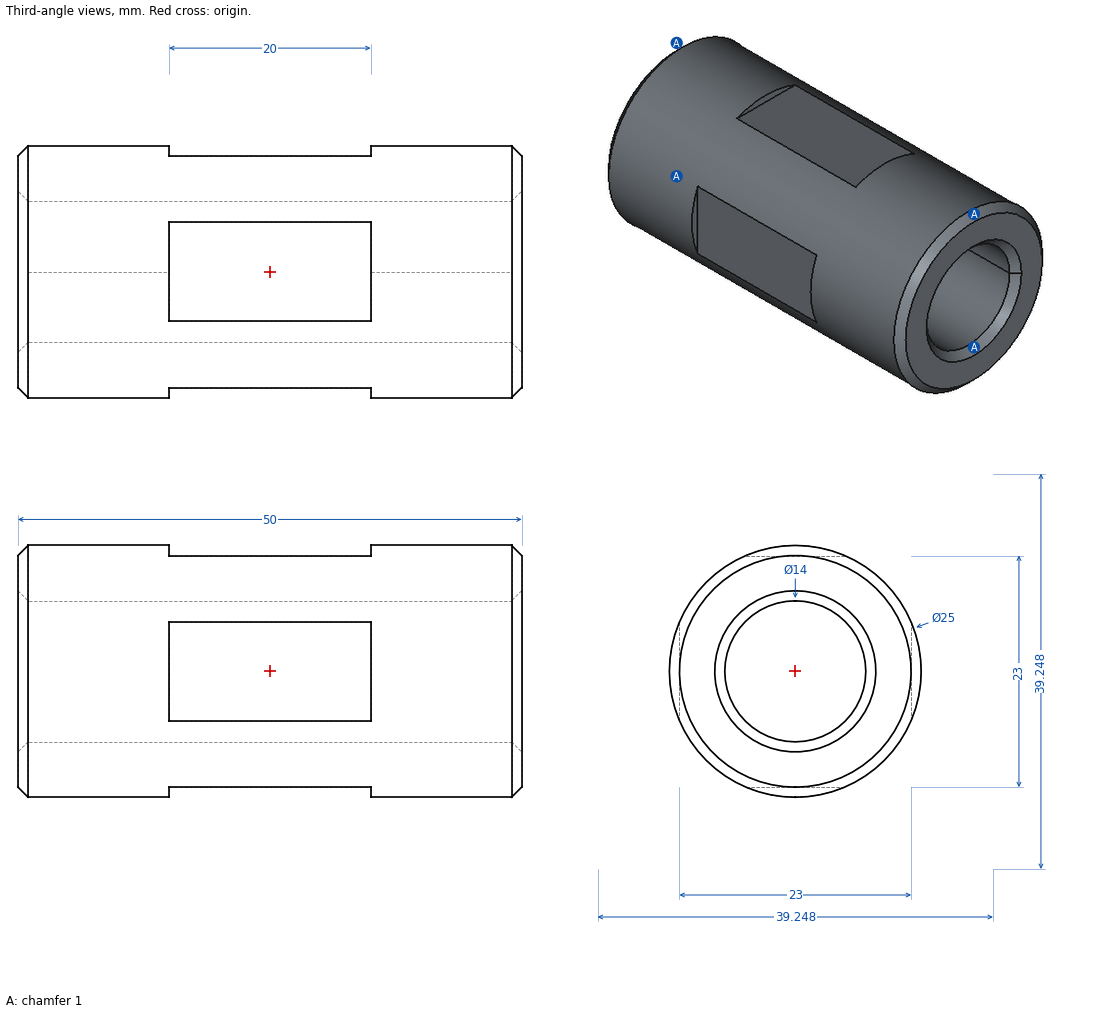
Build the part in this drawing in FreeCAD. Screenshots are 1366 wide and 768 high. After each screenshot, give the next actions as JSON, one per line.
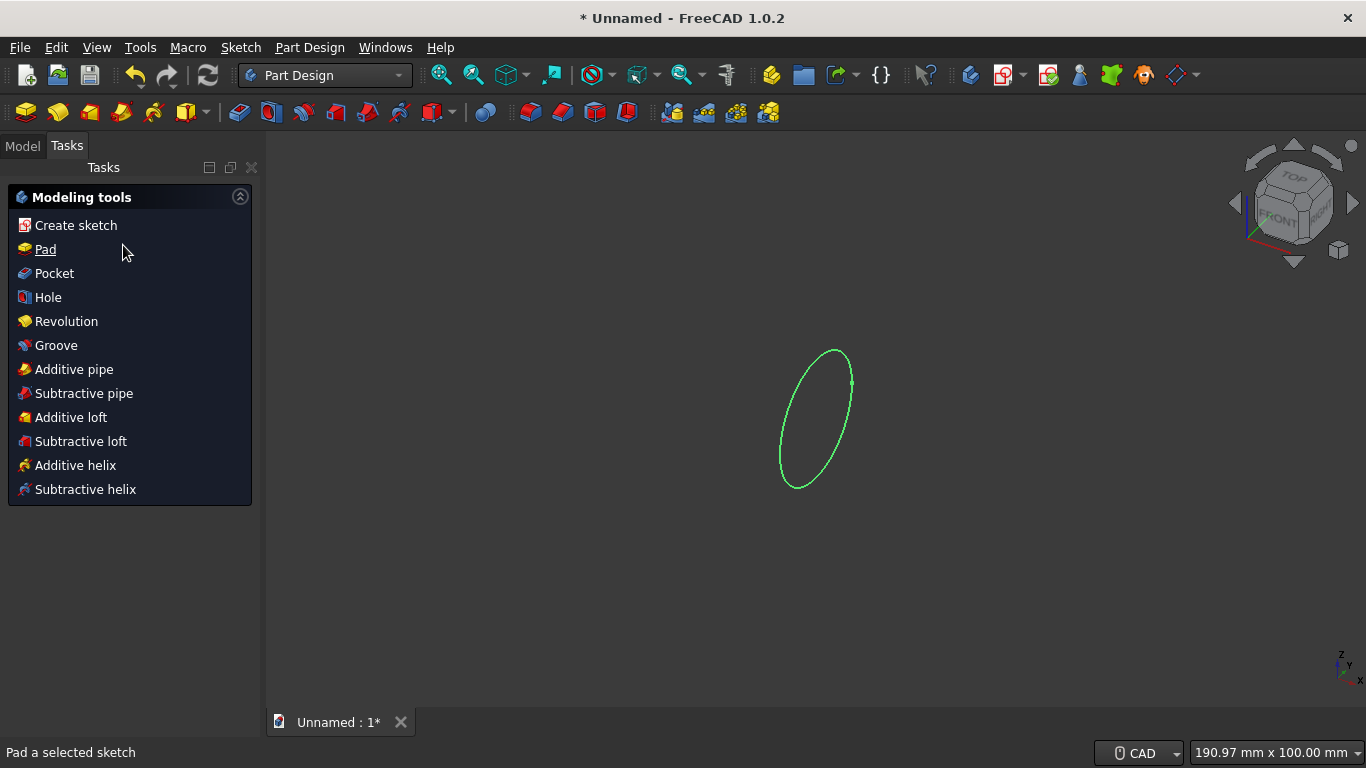
{"action": "left_click", "coordinate": [26, 112]}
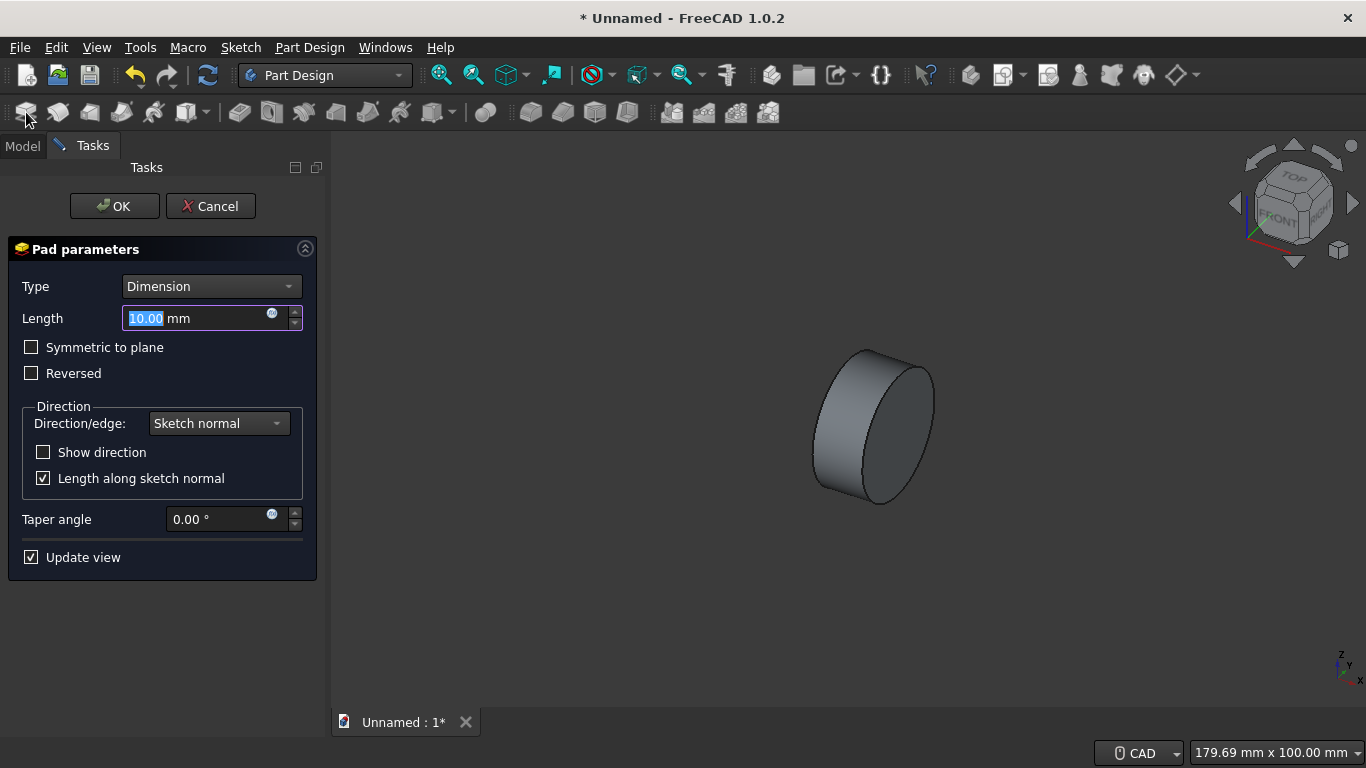
{"action": "type", "text": "50"}
{"action": "key", "text": "Tab"}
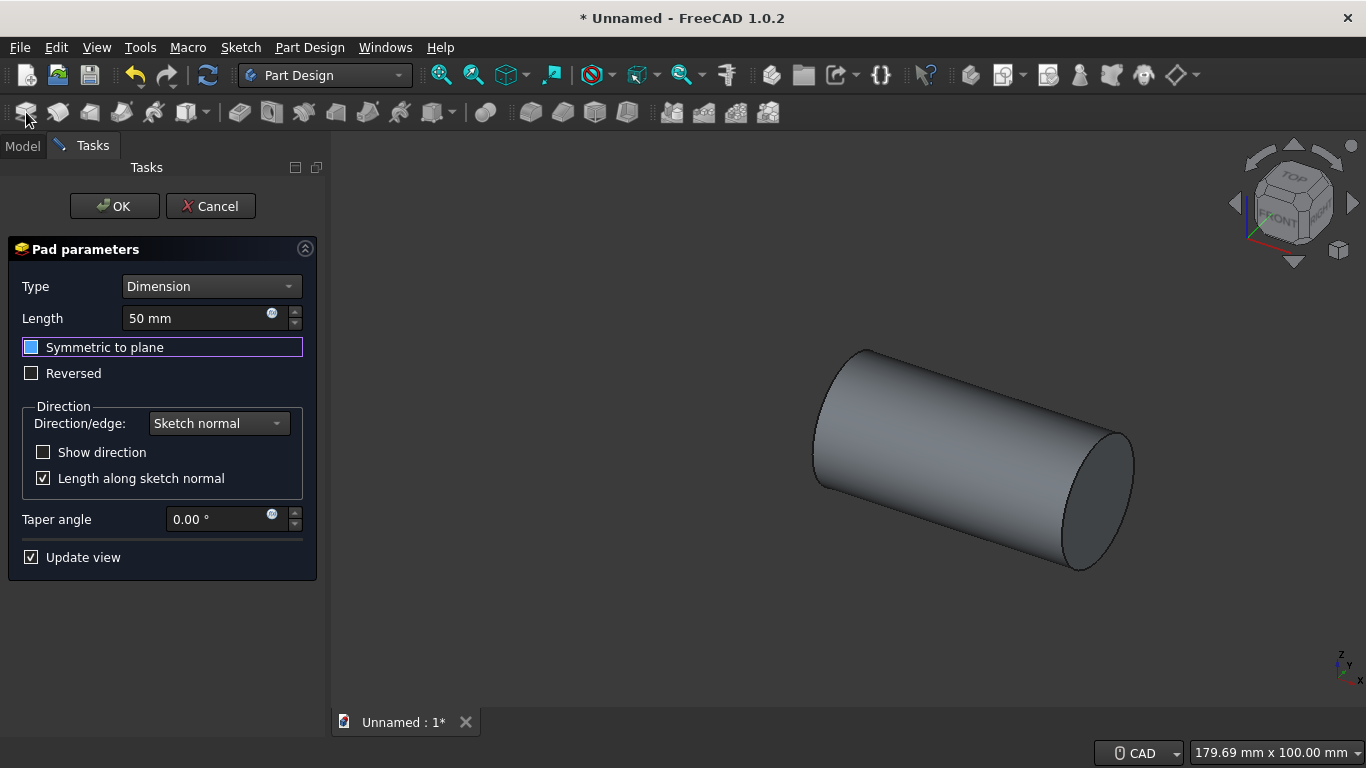
{"action": "left_click", "coordinate": [30, 347]}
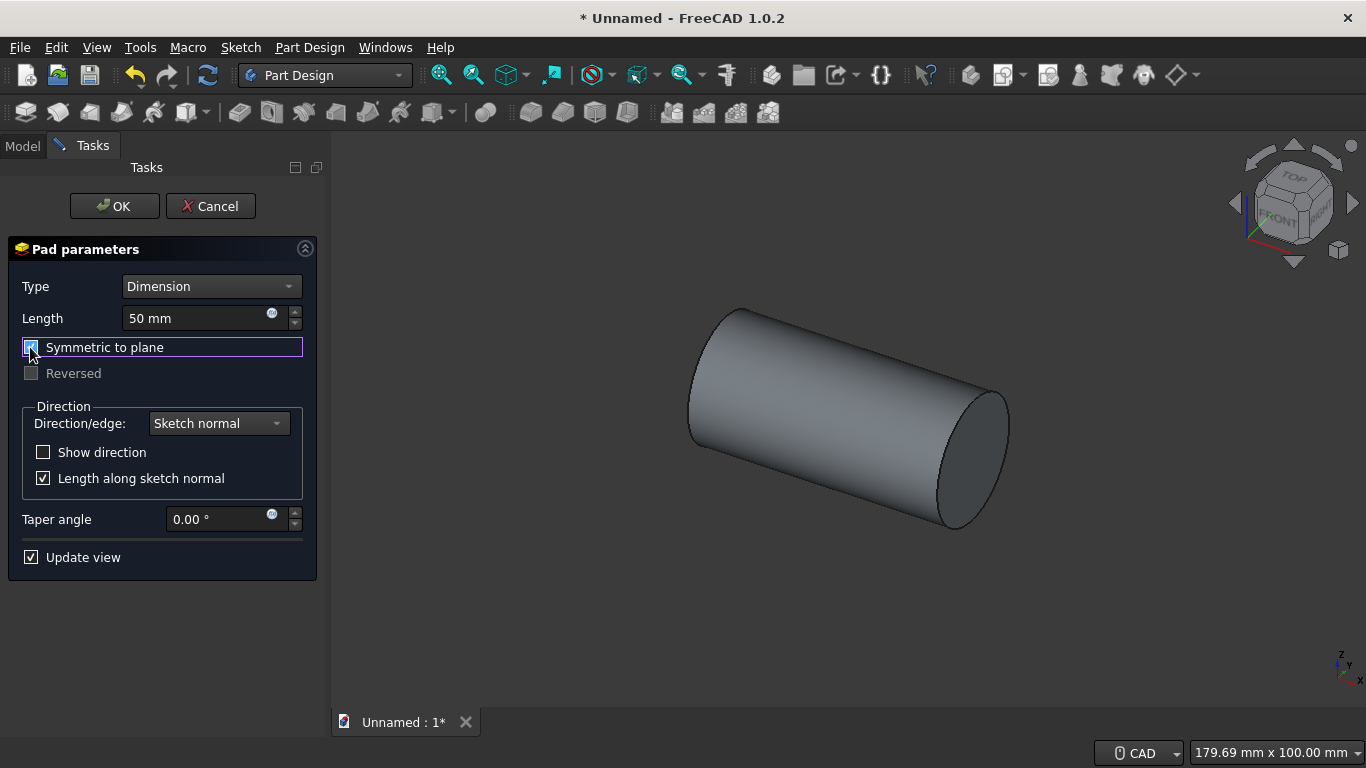
{"action": "left_click", "coordinate": [115, 206]}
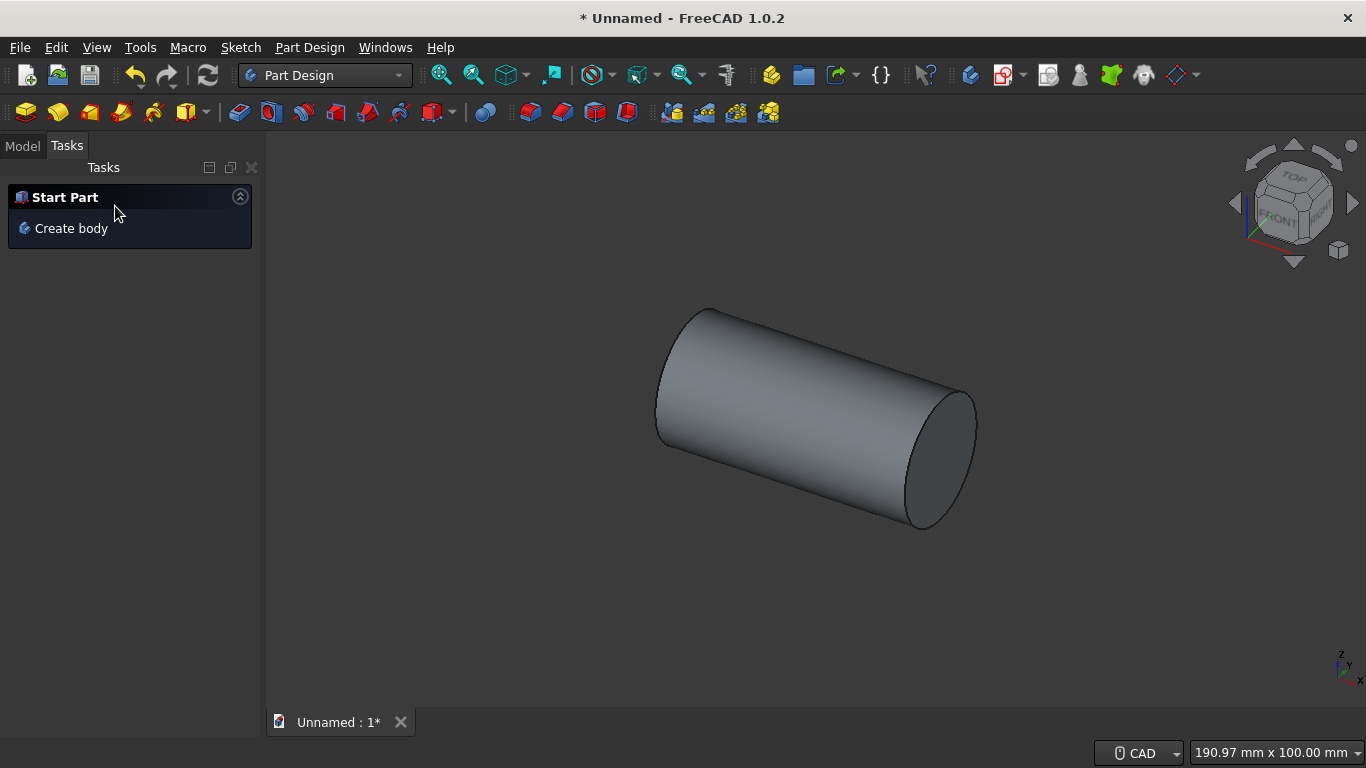
{"action": "left_click", "coordinate": [941, 459]}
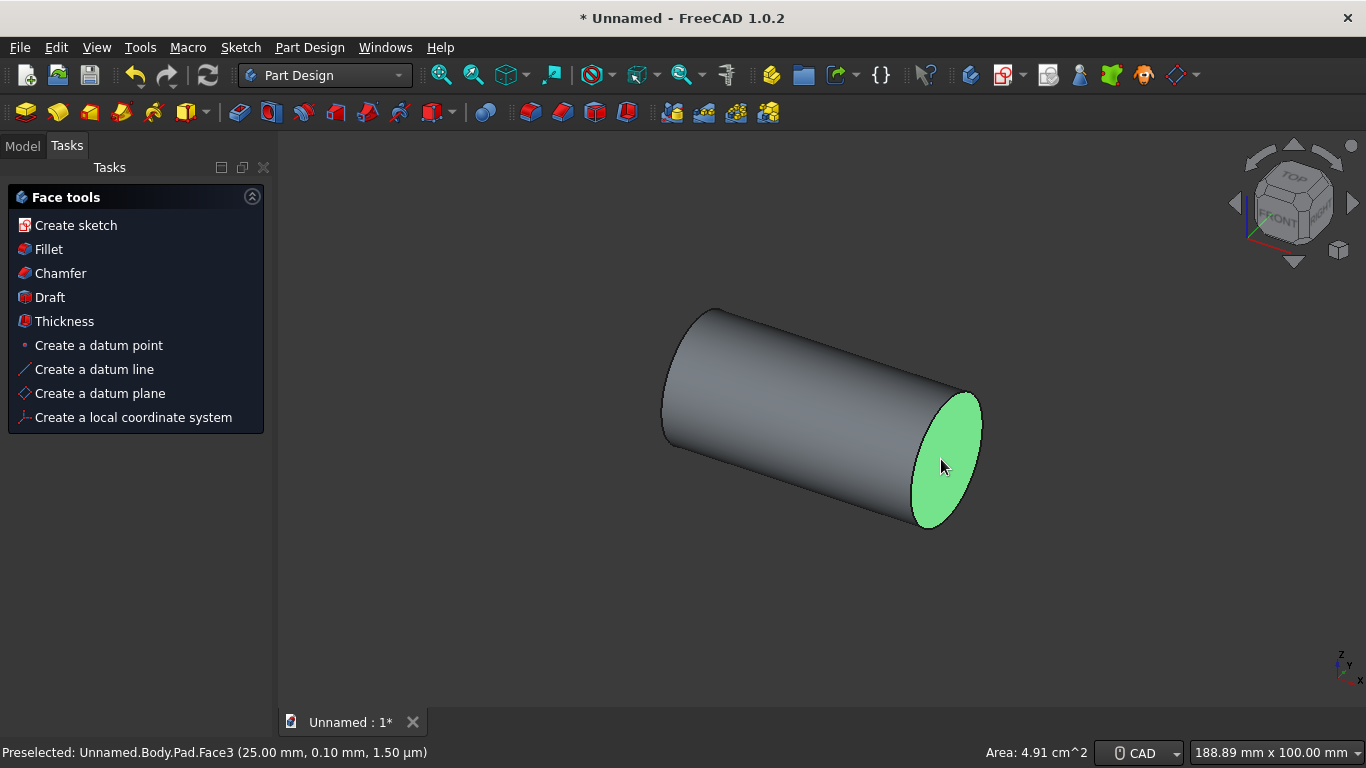
{"action": "left_click", "coordinate": [1004, 76]}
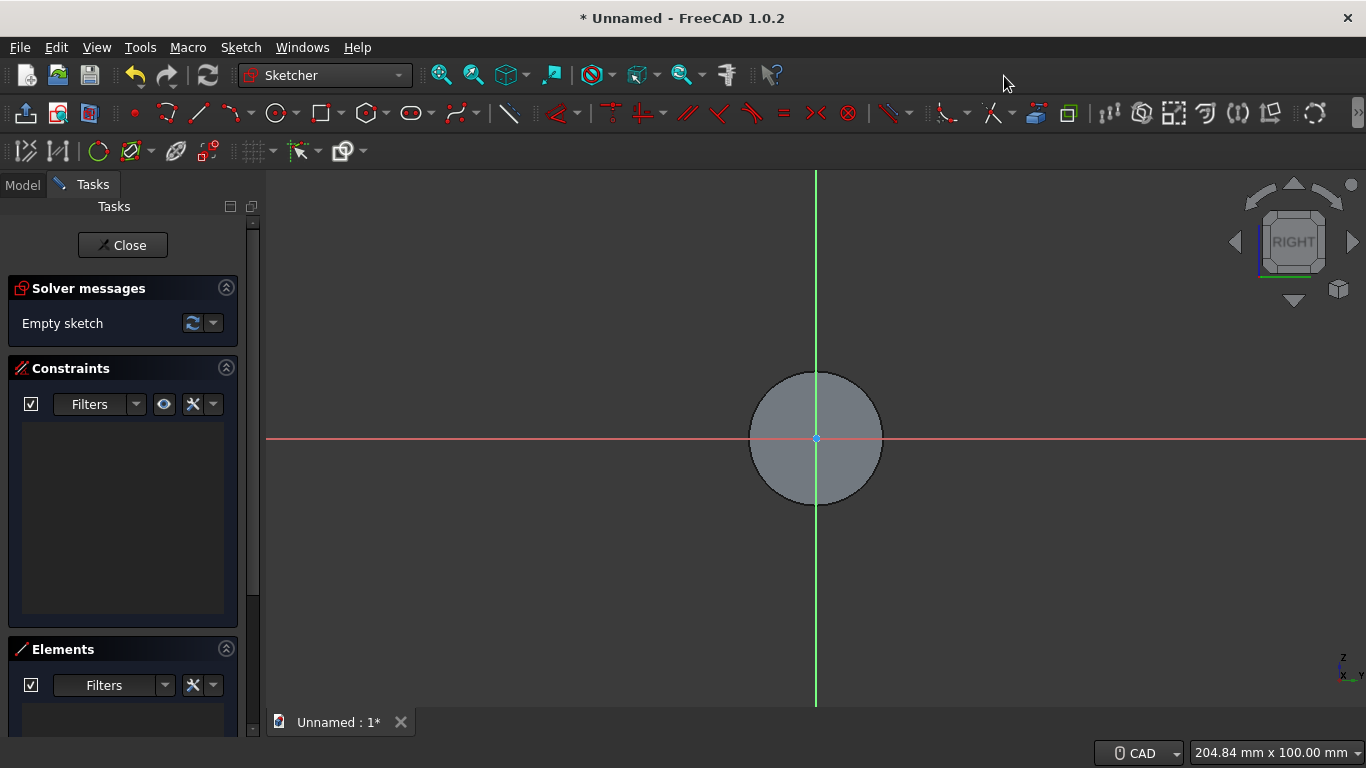
{"action": "scroll", "coordinate": [833, 438], "scroll_direction": "up", "scroll_amount": 8}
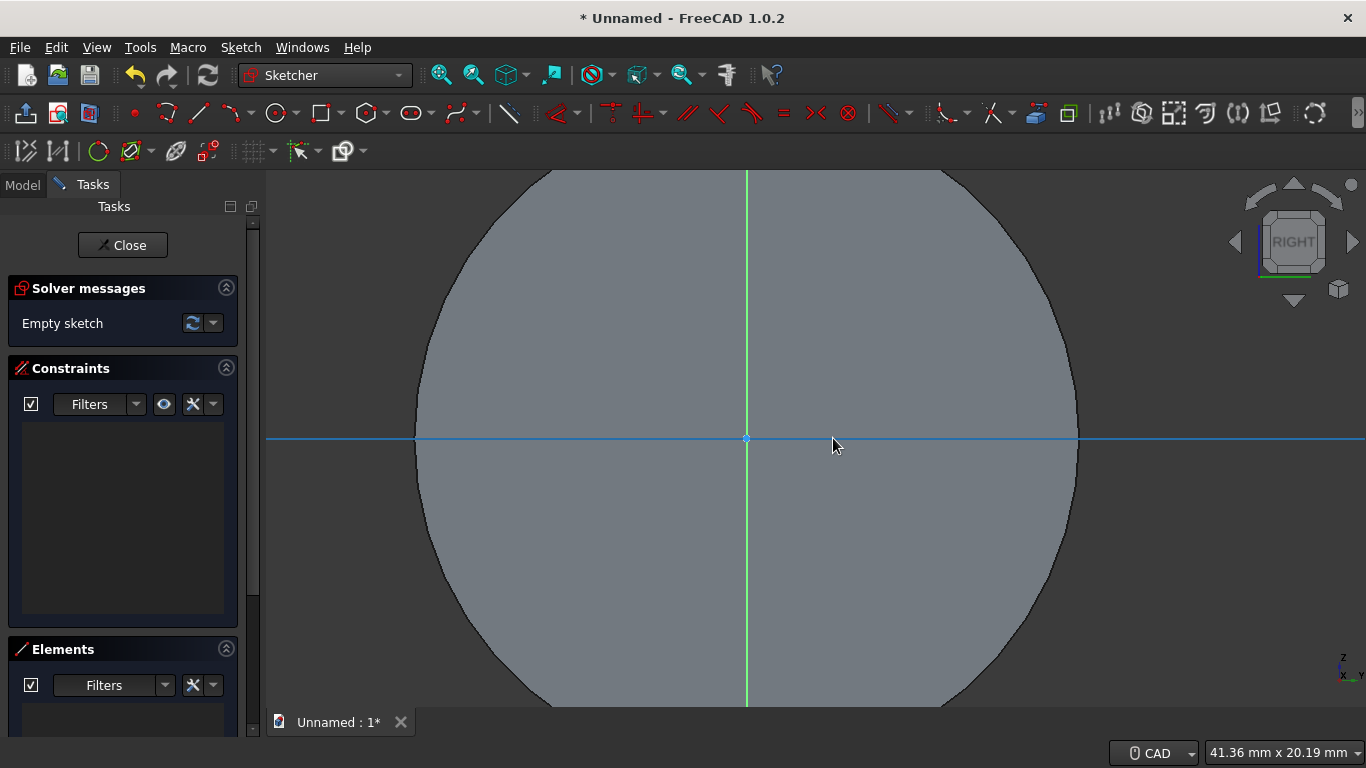
{"action": "left_click", "coordinate": [276, 114]}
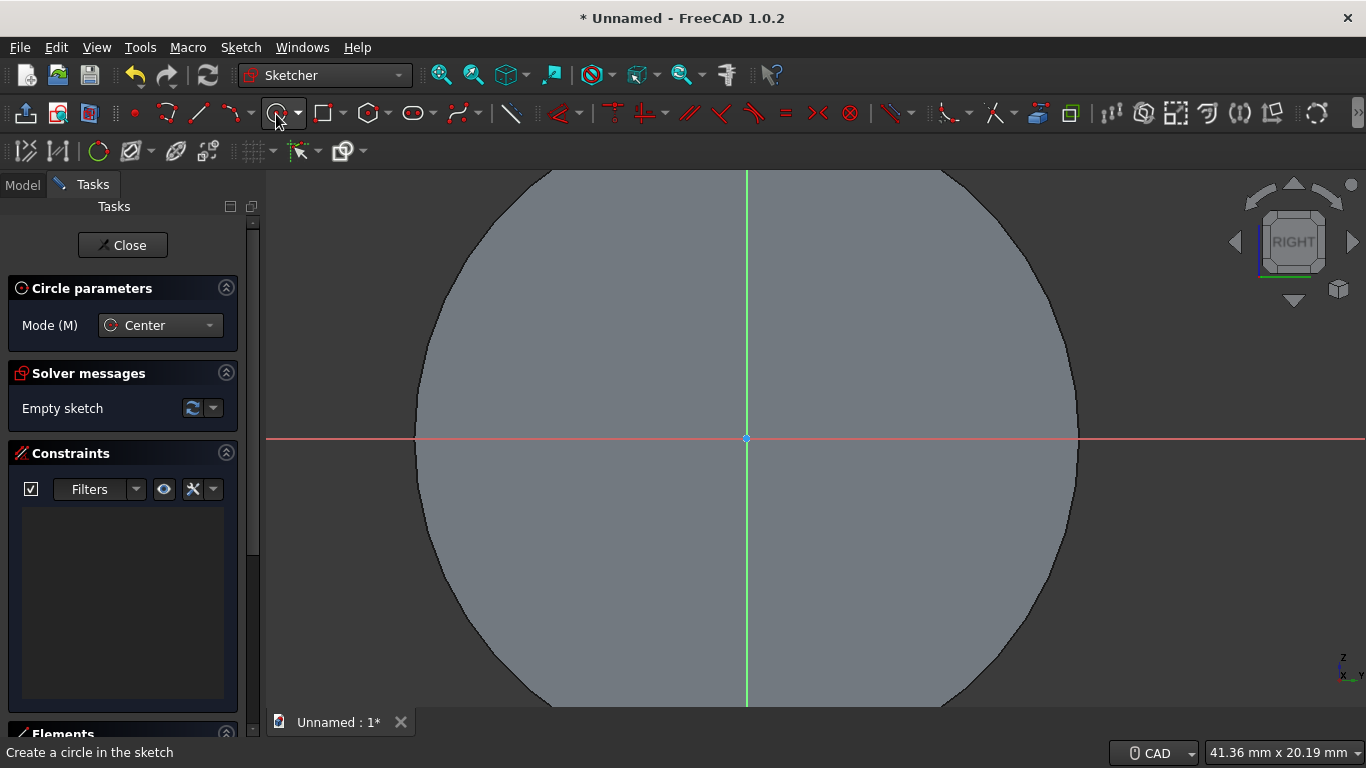
{"action": "left_click", "coordinate": [747, 438]}
{"action": "mouse_move", "coordinate": [878, 307]}